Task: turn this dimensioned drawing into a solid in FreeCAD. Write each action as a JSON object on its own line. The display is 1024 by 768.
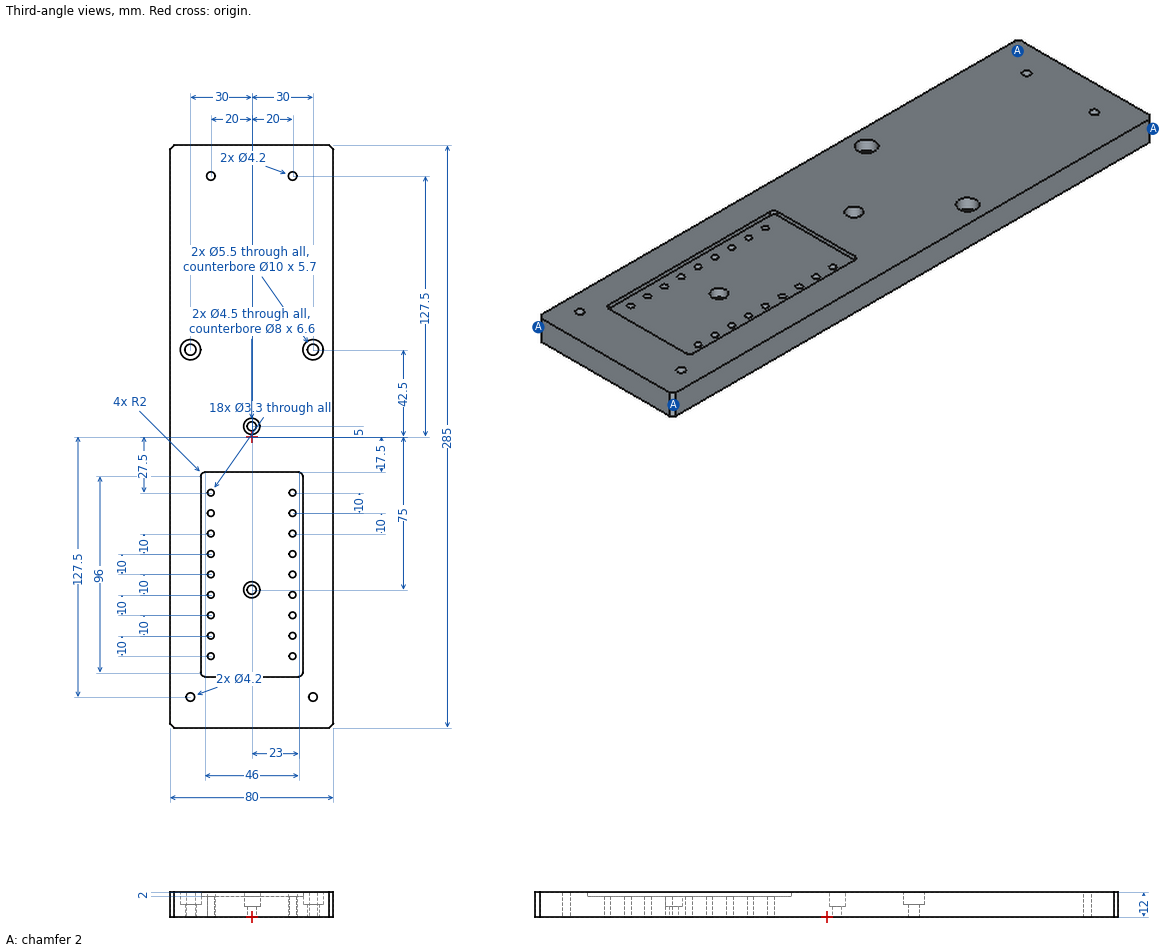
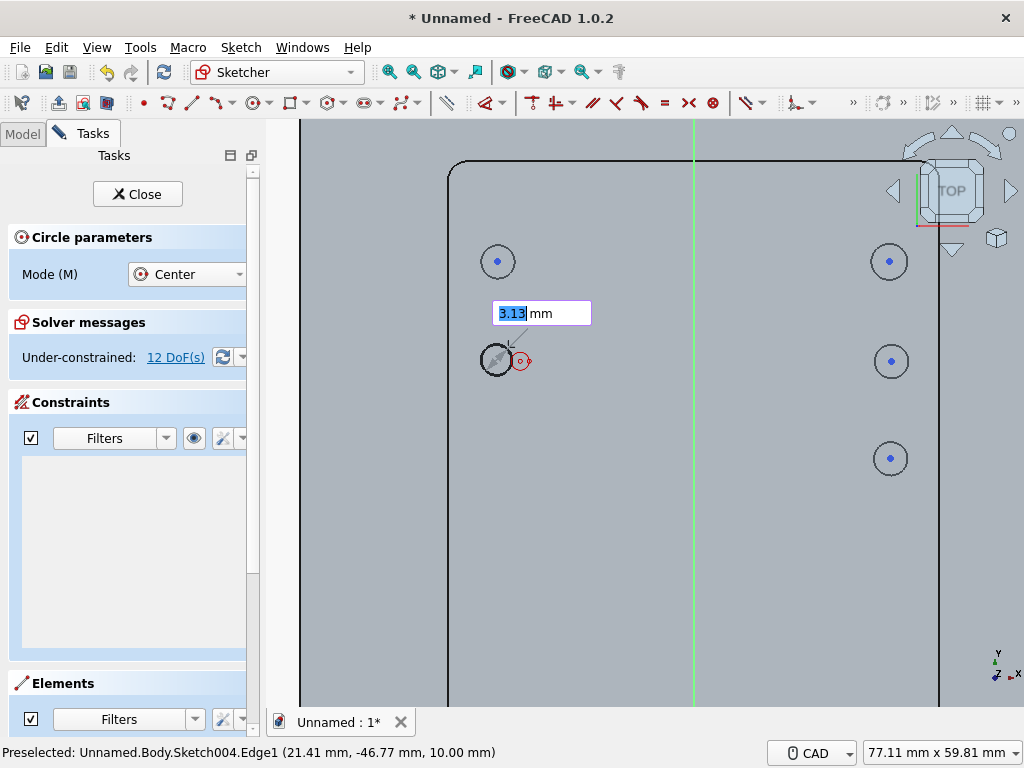
{"action": "left_click", "coordinate": [509, 346]}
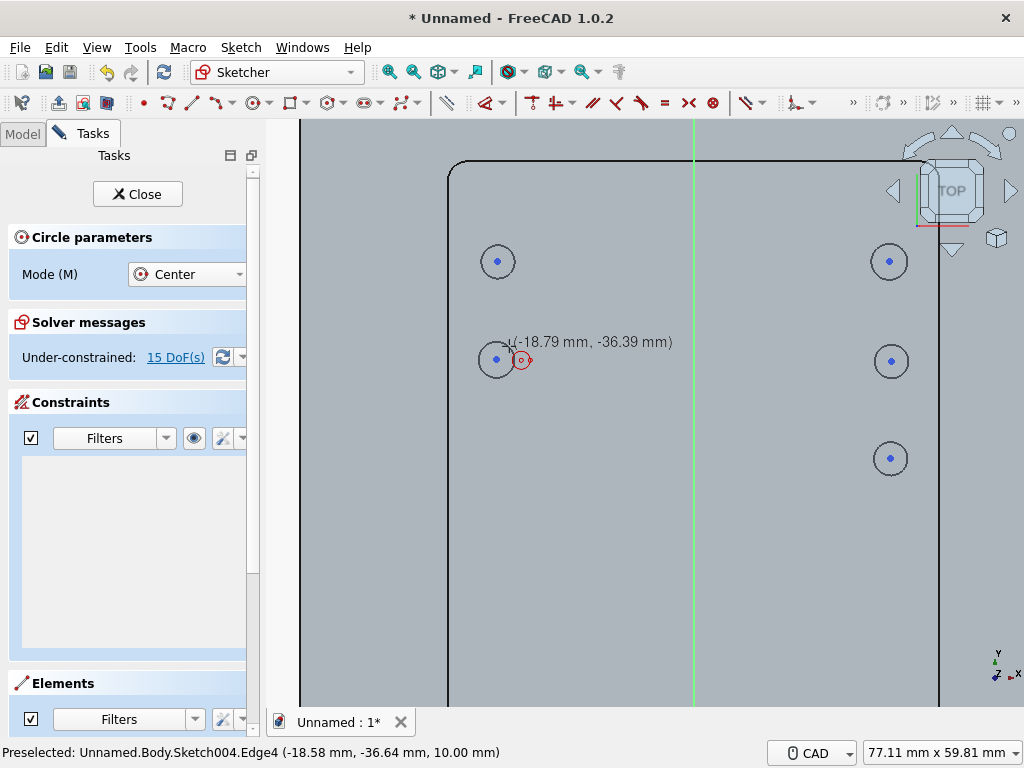
{"action": "scroll", "coordinate": [497, 456], "scroll_direction": "up", "scroll_amount": 2}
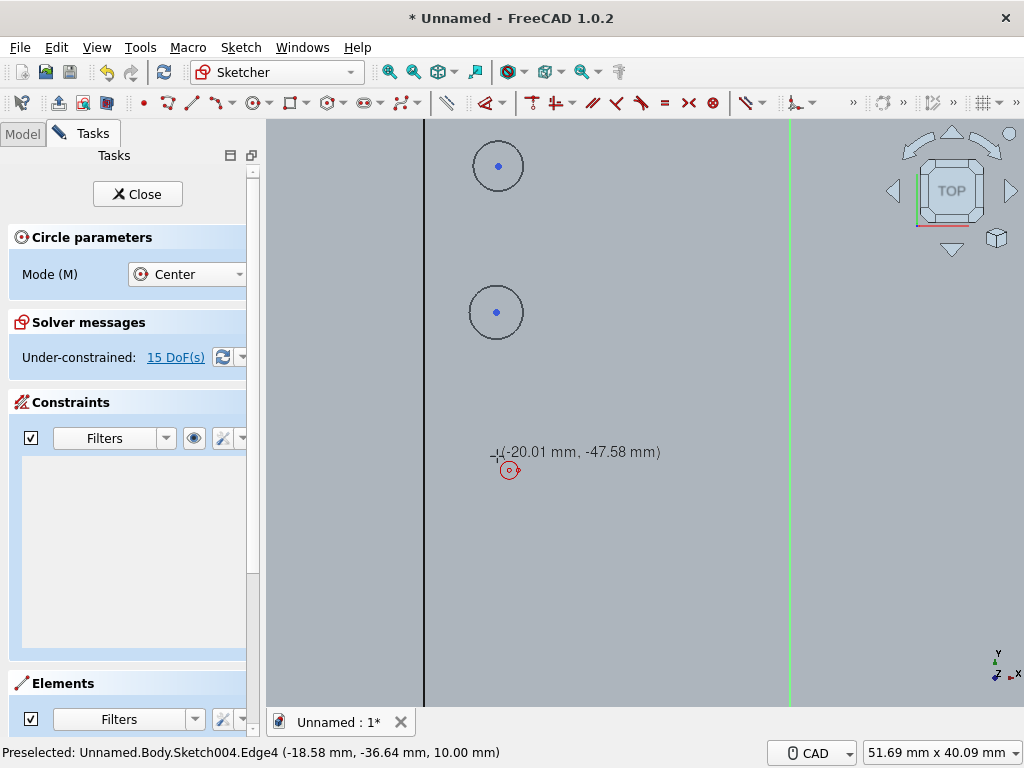
{"action": "scroll", "coordinate": [507, 365], "scroll_direction": "down", "scroll_amount": 7}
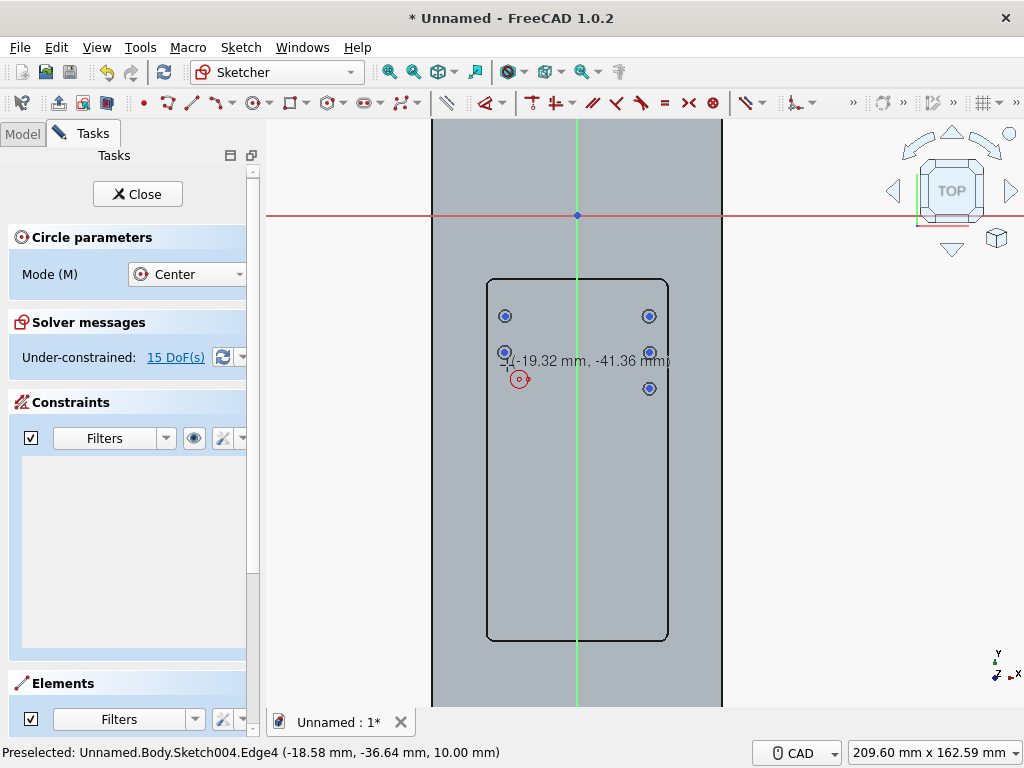
{"action": "left_click", "coordinate": [505, 388]}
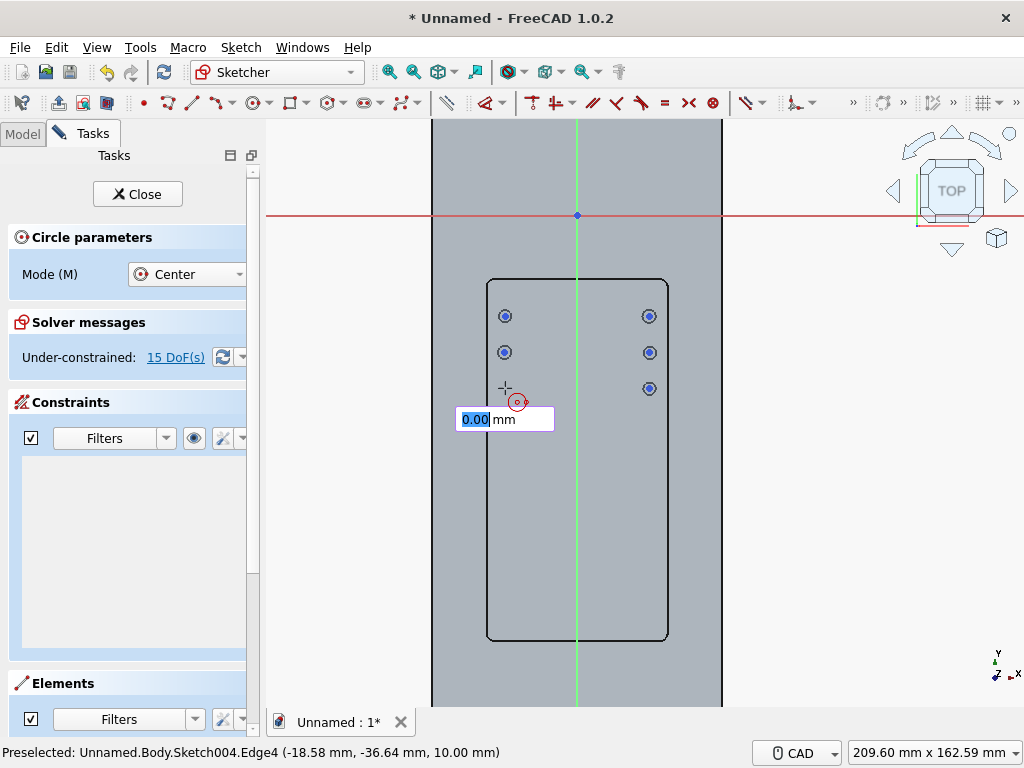
{"action": "scroll", "coordinate": [509, 384], "scroll_direction": "up", "scroll_amount": 5}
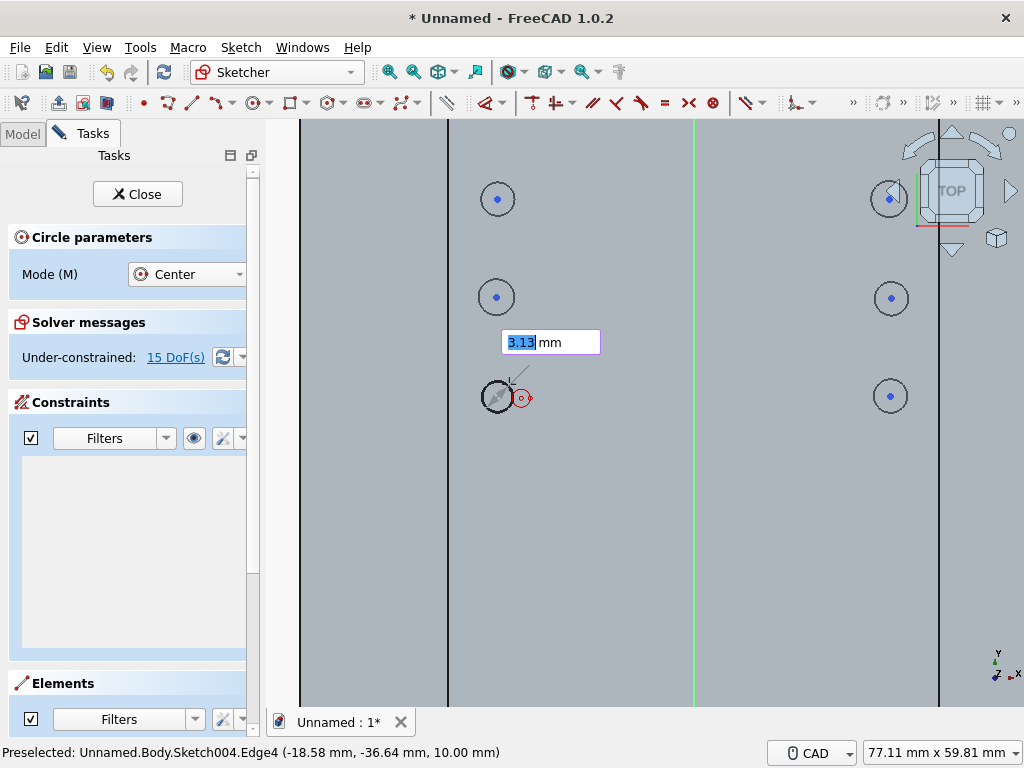
{"action": "left_click", "coordinate": [508, 382]}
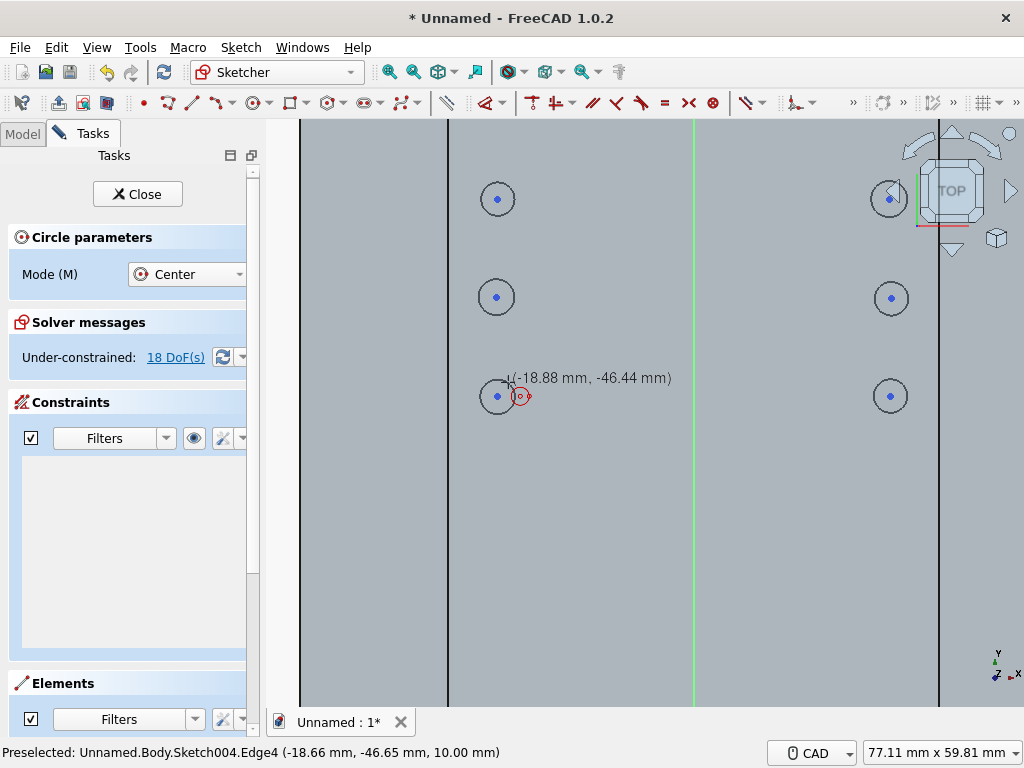
{"action": "scroll", "coordinate": [497, 492], "scroll_direction": "up", "scroll_amount": 2}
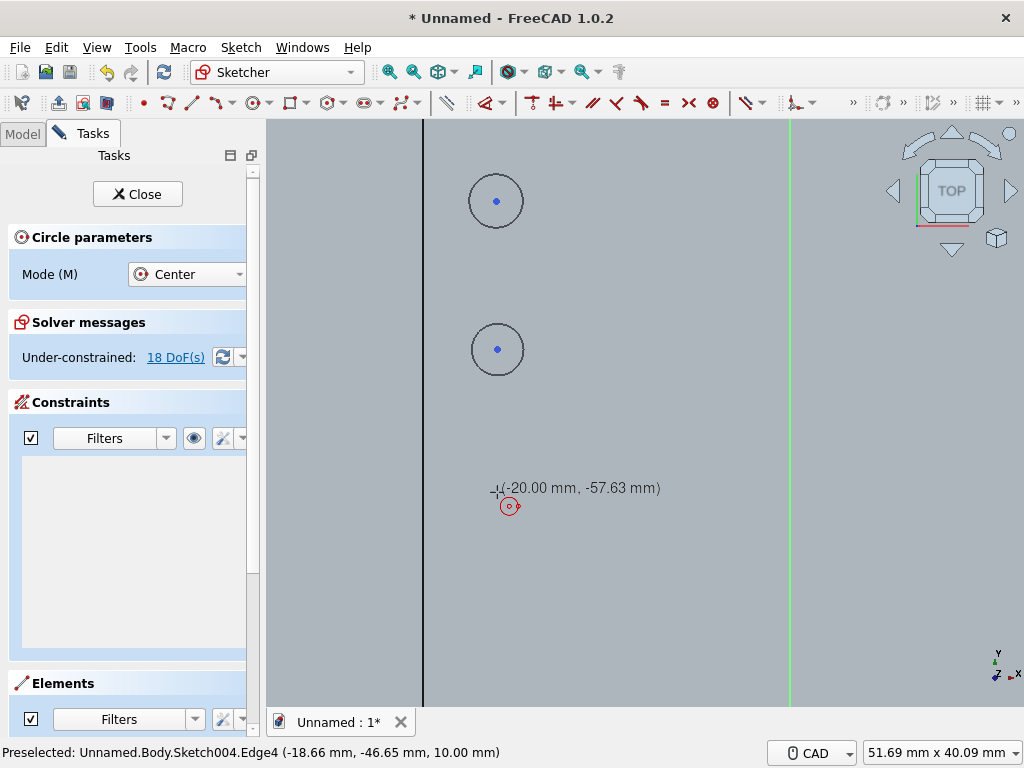
{"action": "scroll", "coordinate": [507, 401], "scroll_direction": "down", "scroll_amount": 7}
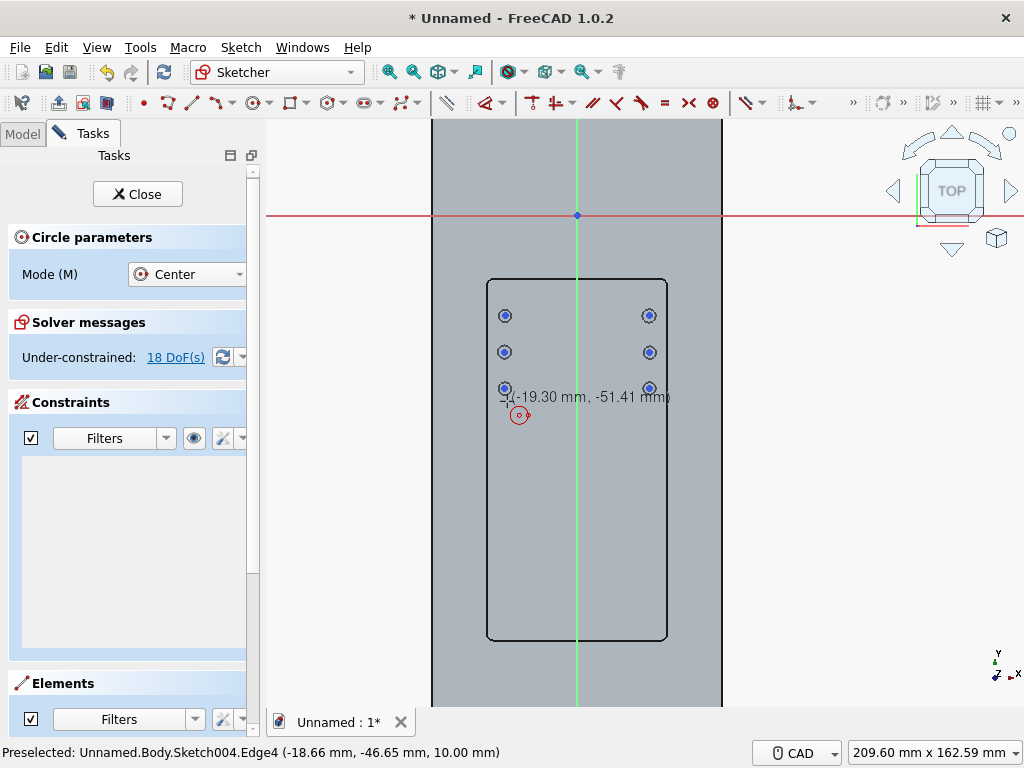
{"action": "left_click", "coordinate": [505, 424]}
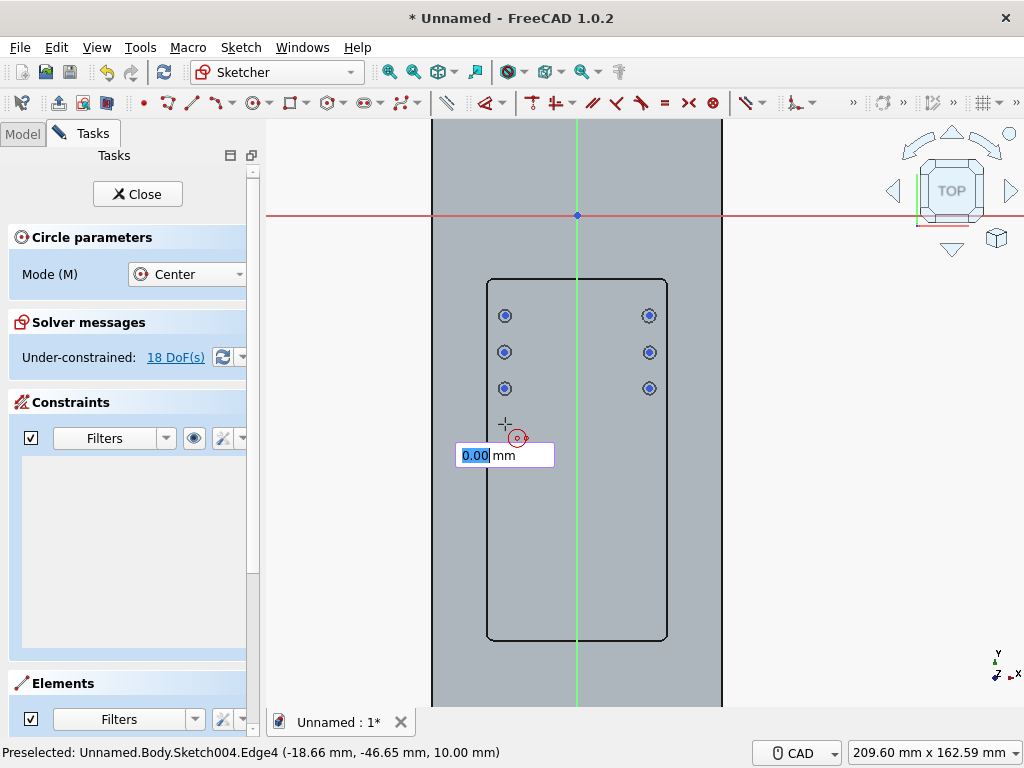
{"action": "scroll", "coordinate": [509, 419], "scroll_direction": "up", "scroll_amount": 5}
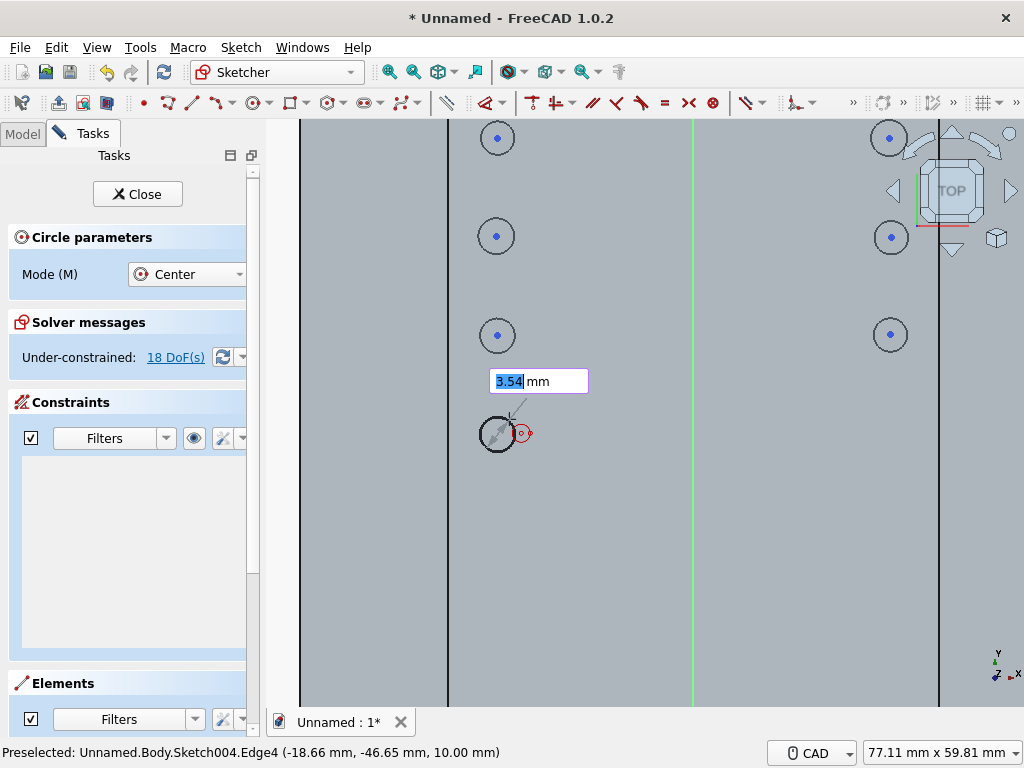
{"action": "left_click", "coordinate": [508, 419]}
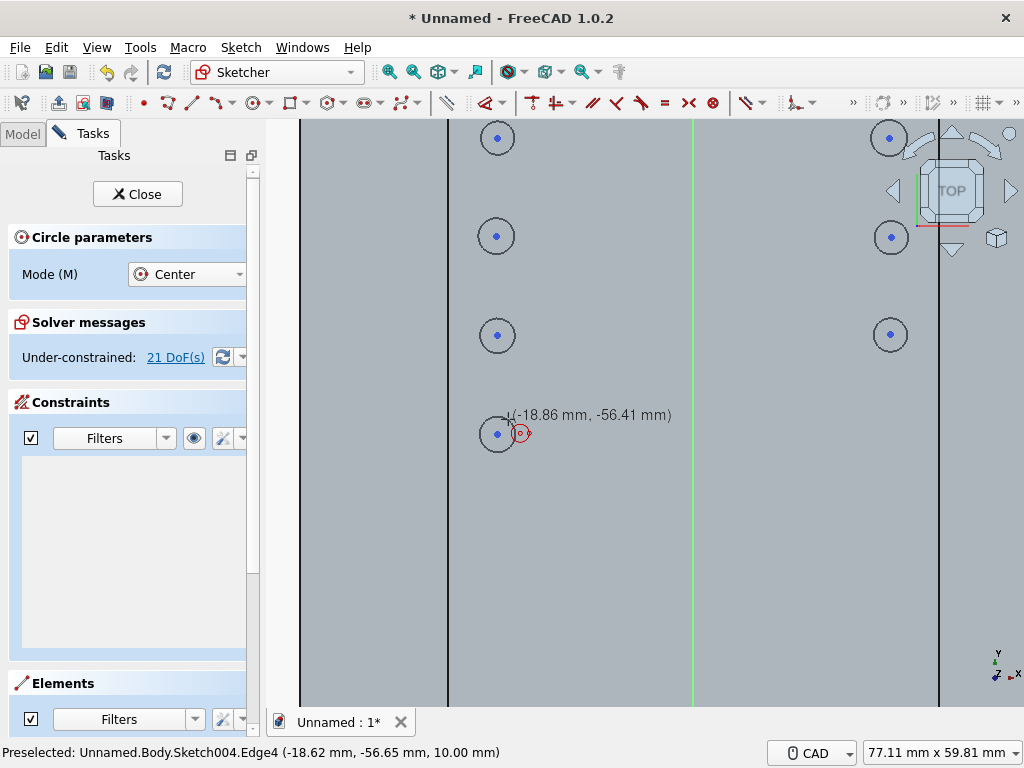
{"action": "scroll", "coordinate": [508, 419], "scroll_direction": "down", "scroll_amount": 5}